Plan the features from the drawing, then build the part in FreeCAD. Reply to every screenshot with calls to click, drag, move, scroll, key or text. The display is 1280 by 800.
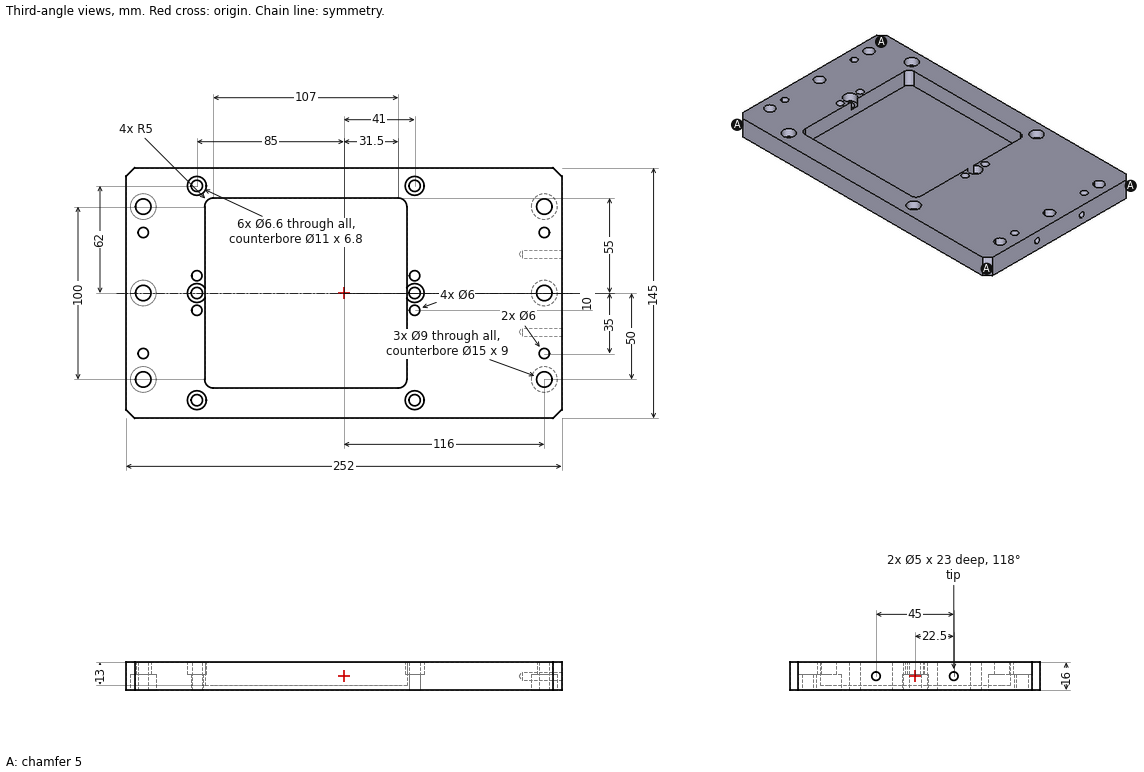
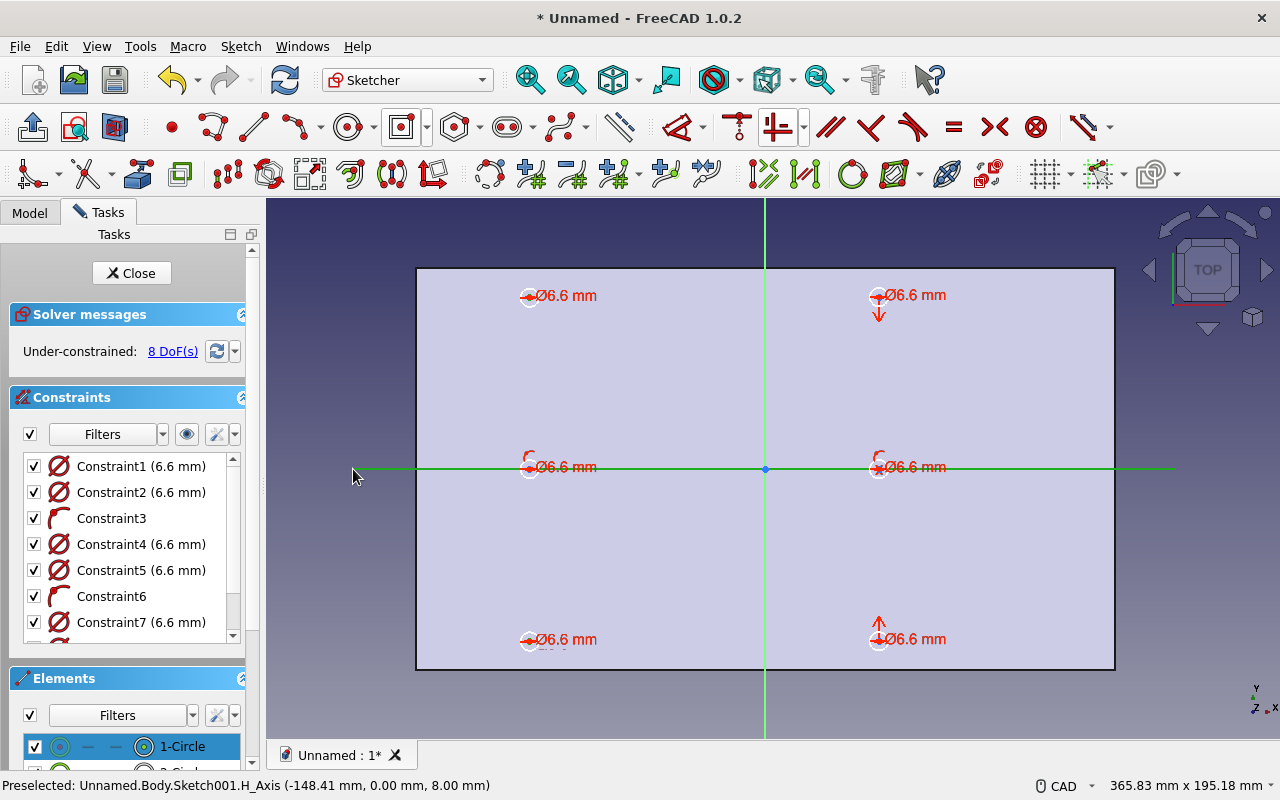
key(s)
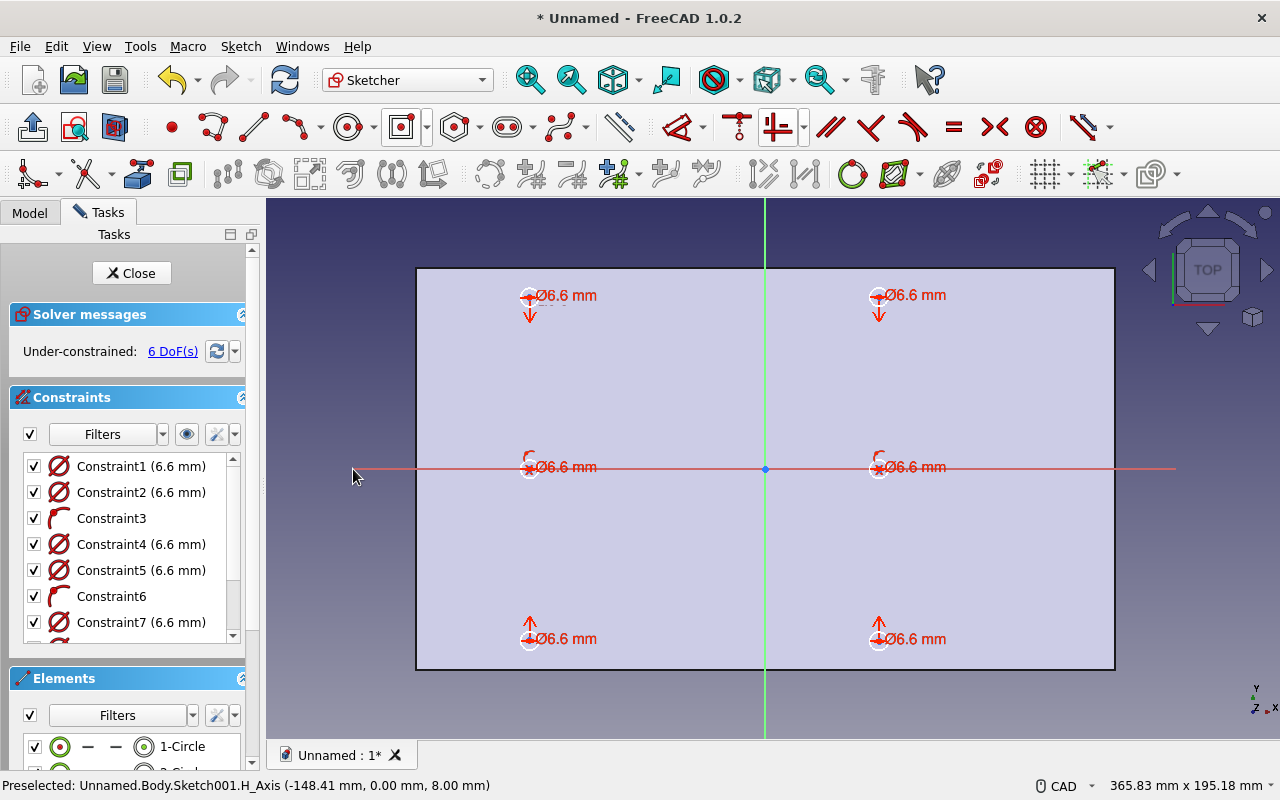
key(d)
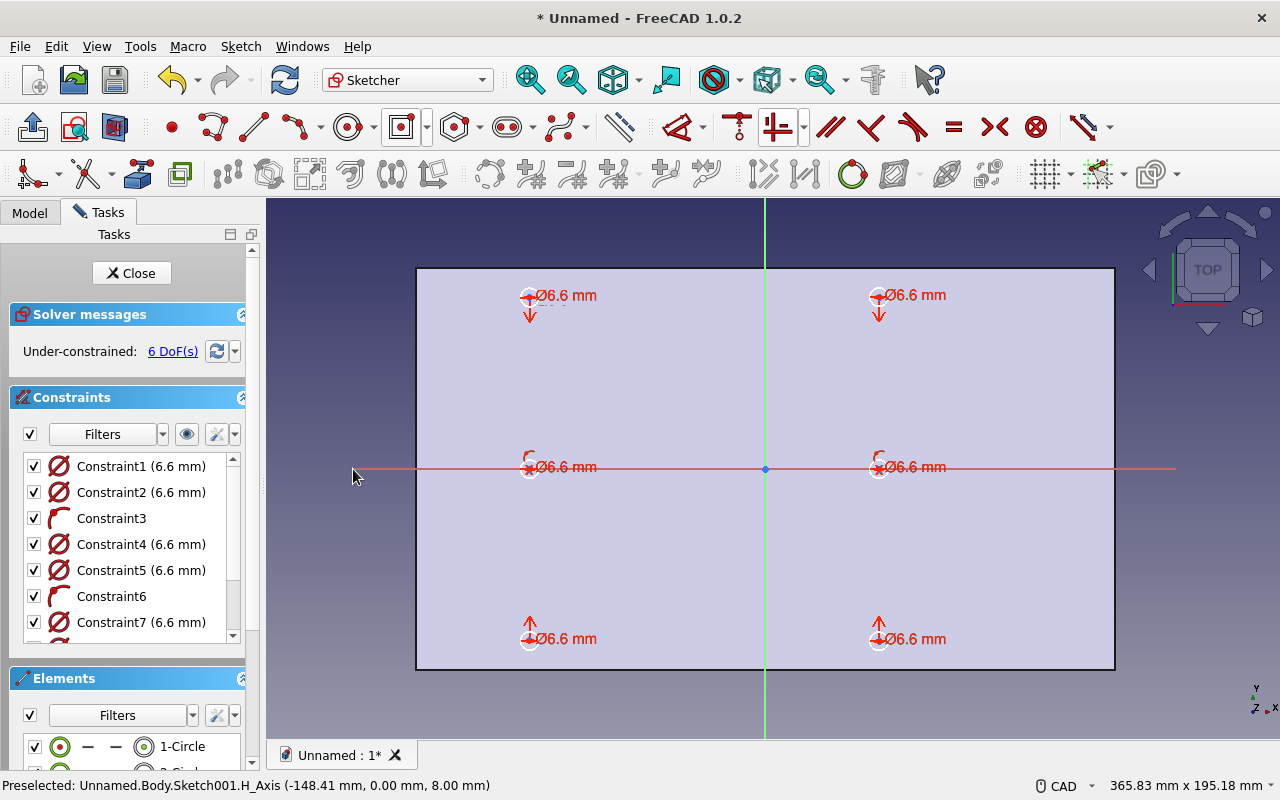
click(530, 298)
click(648, 264)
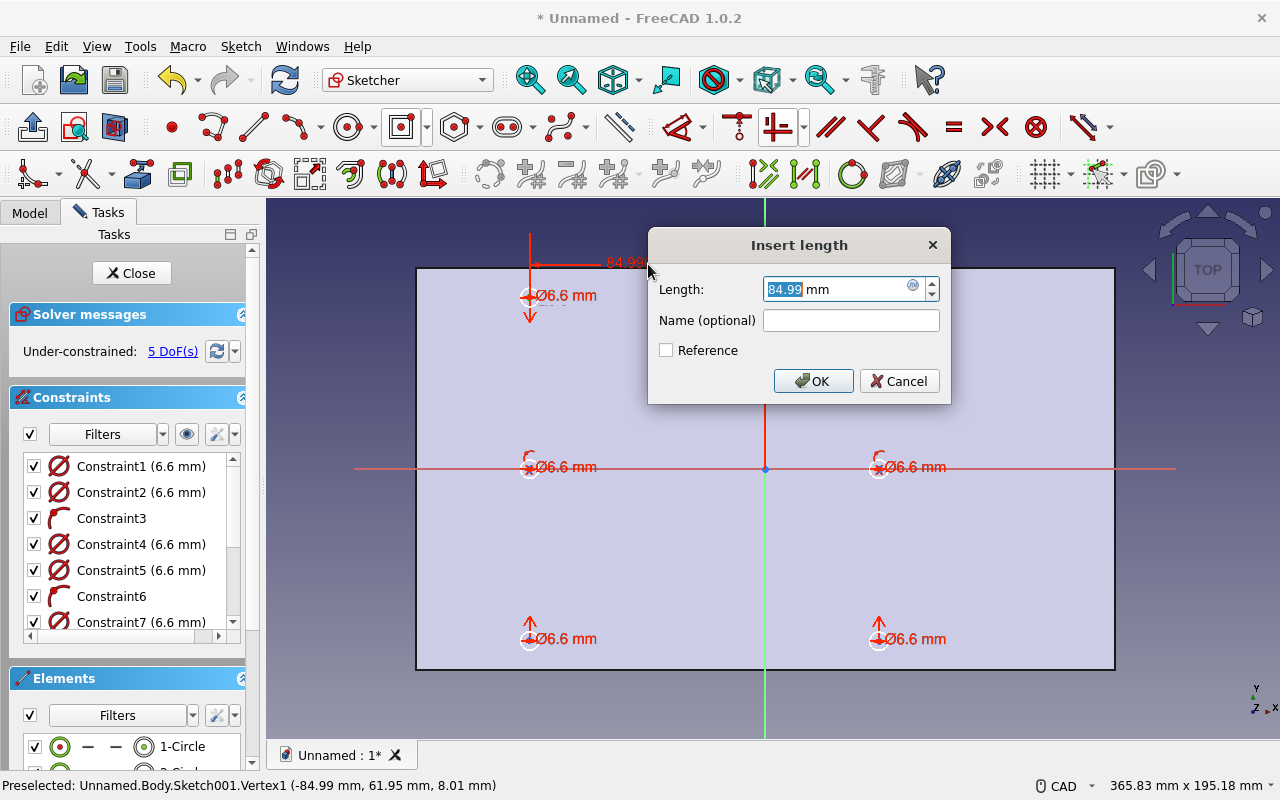
text(85)
key(Return)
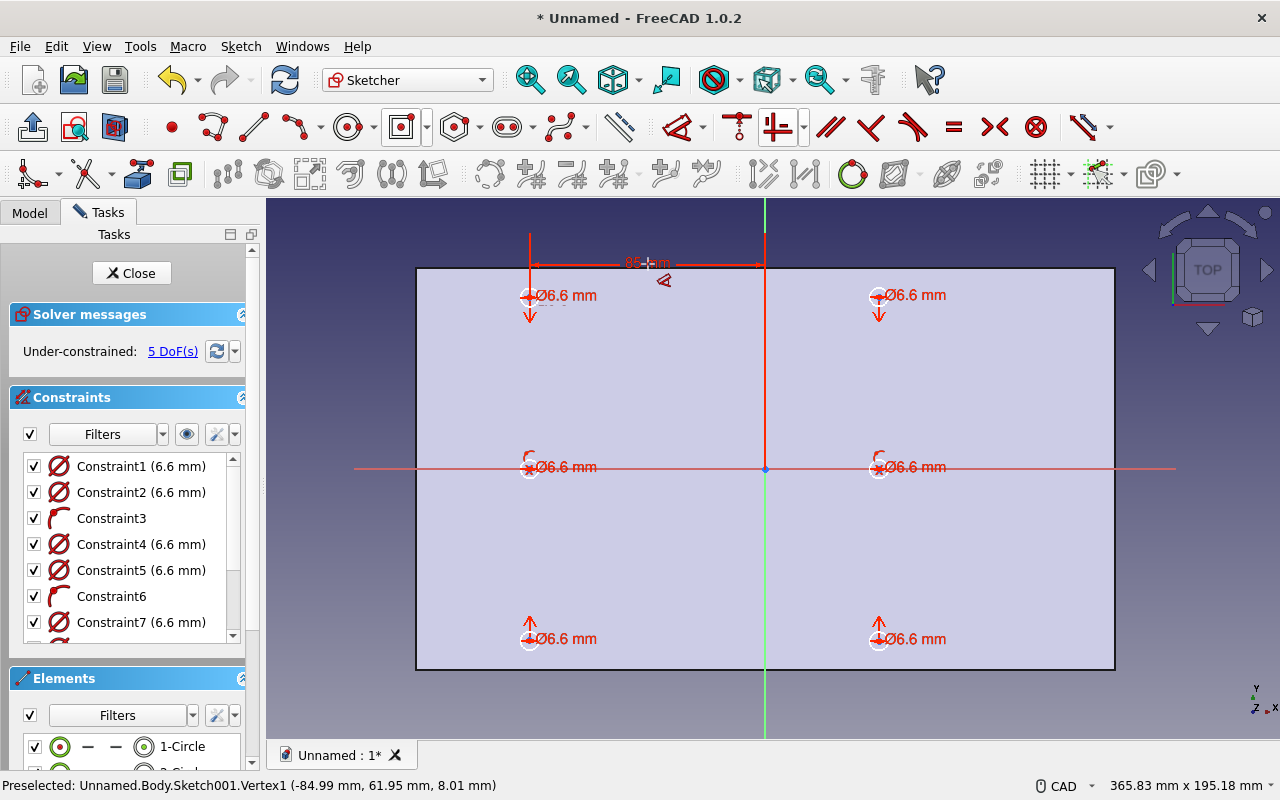
click(530, 298)
click(496, 383)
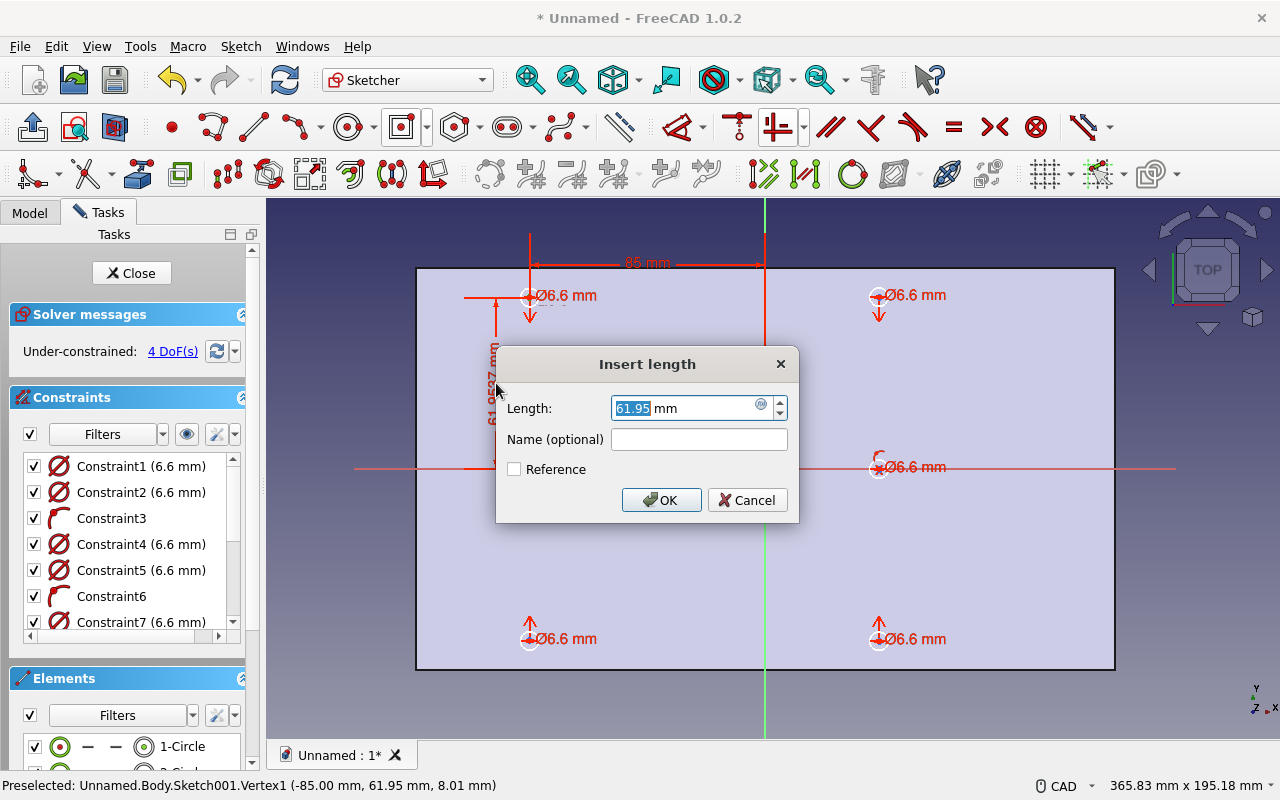
text(62)
key(Return)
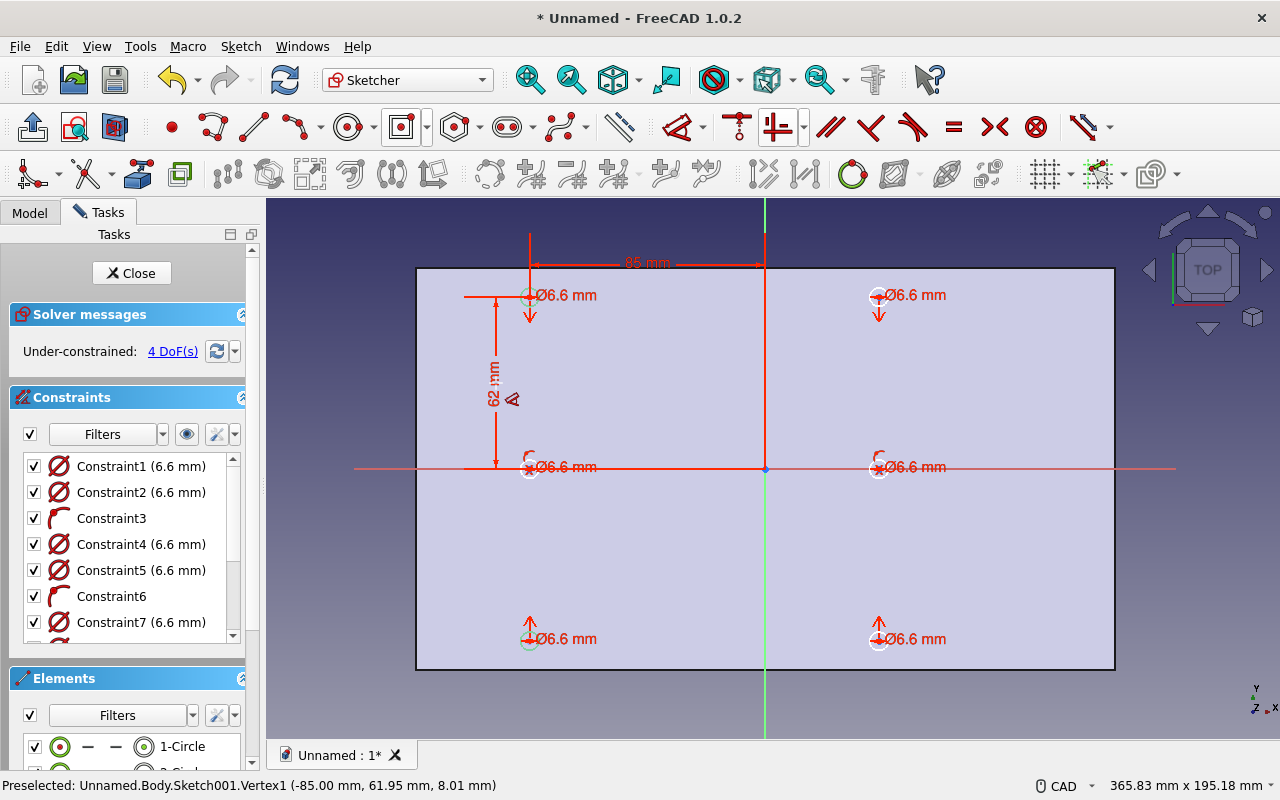
click(530, 469)
click(648, 503)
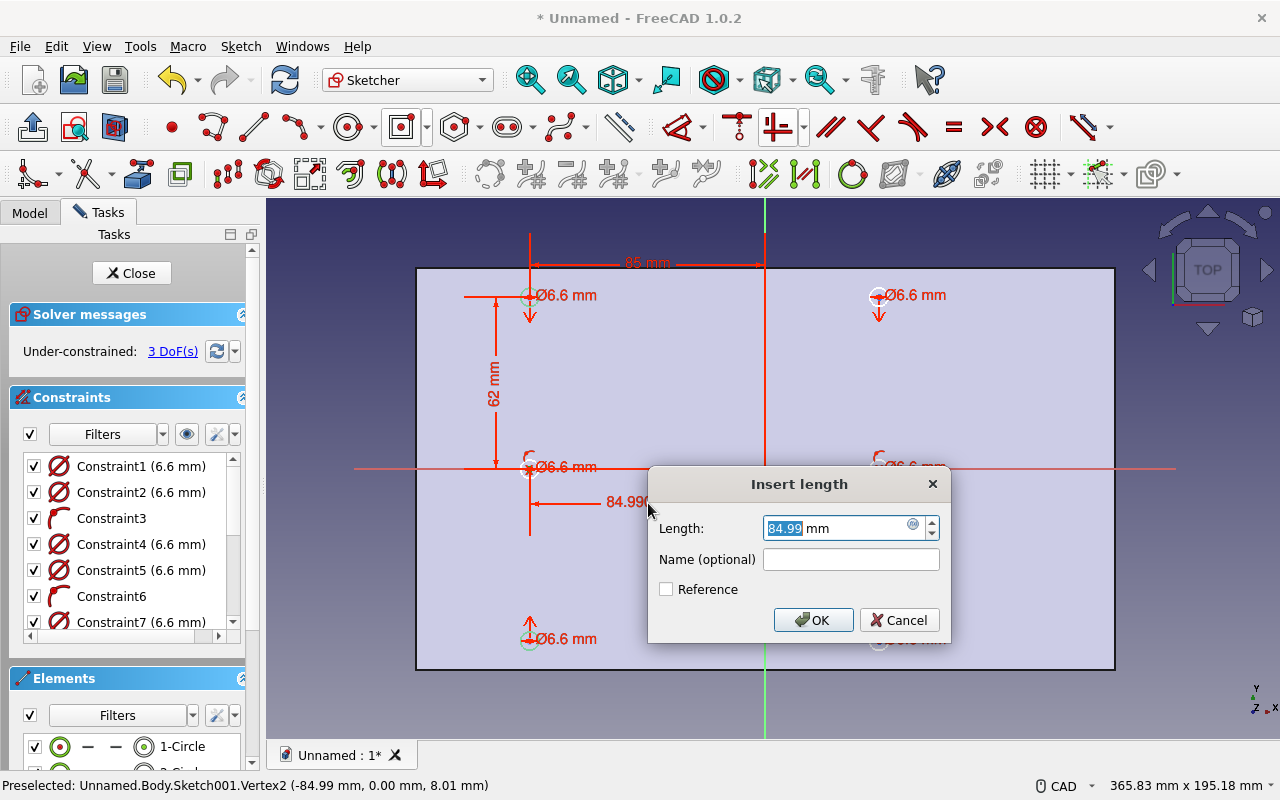
text(85)
key(Return)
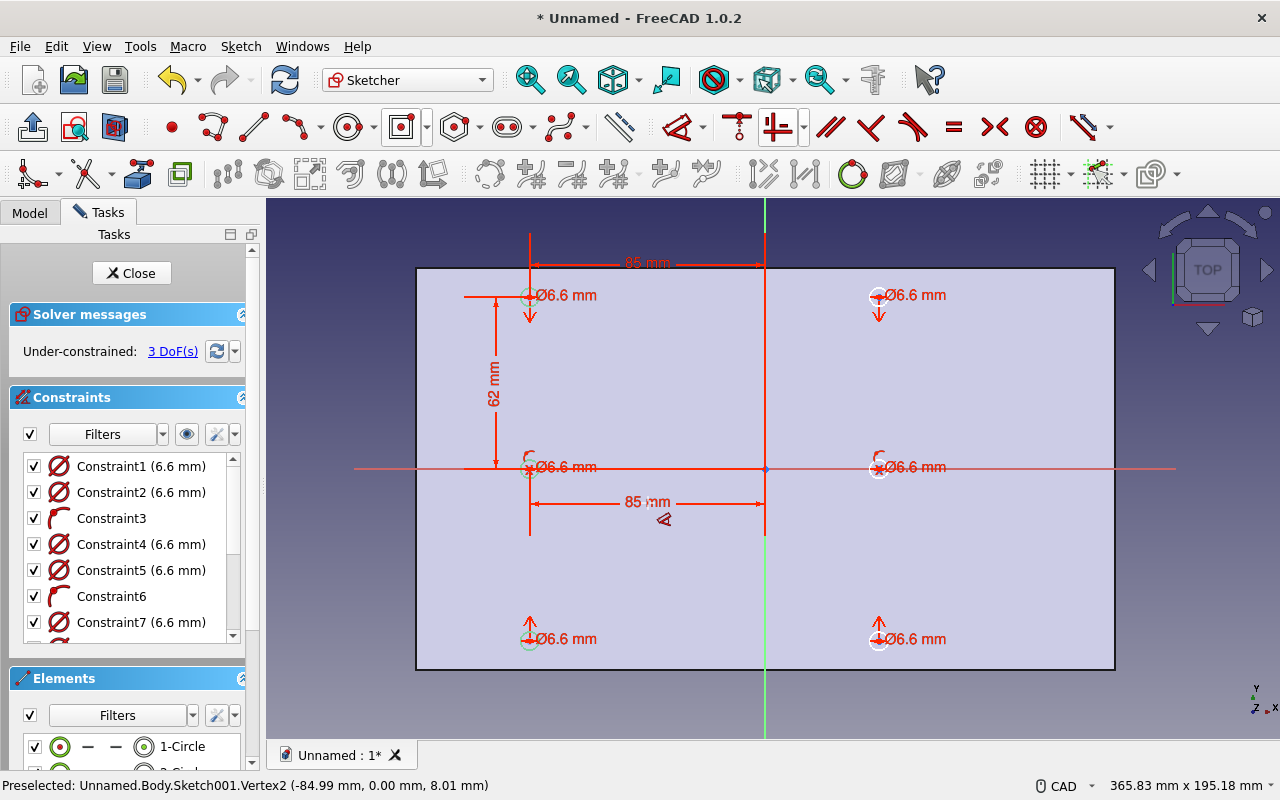
click(879, 297)
click(822, 263)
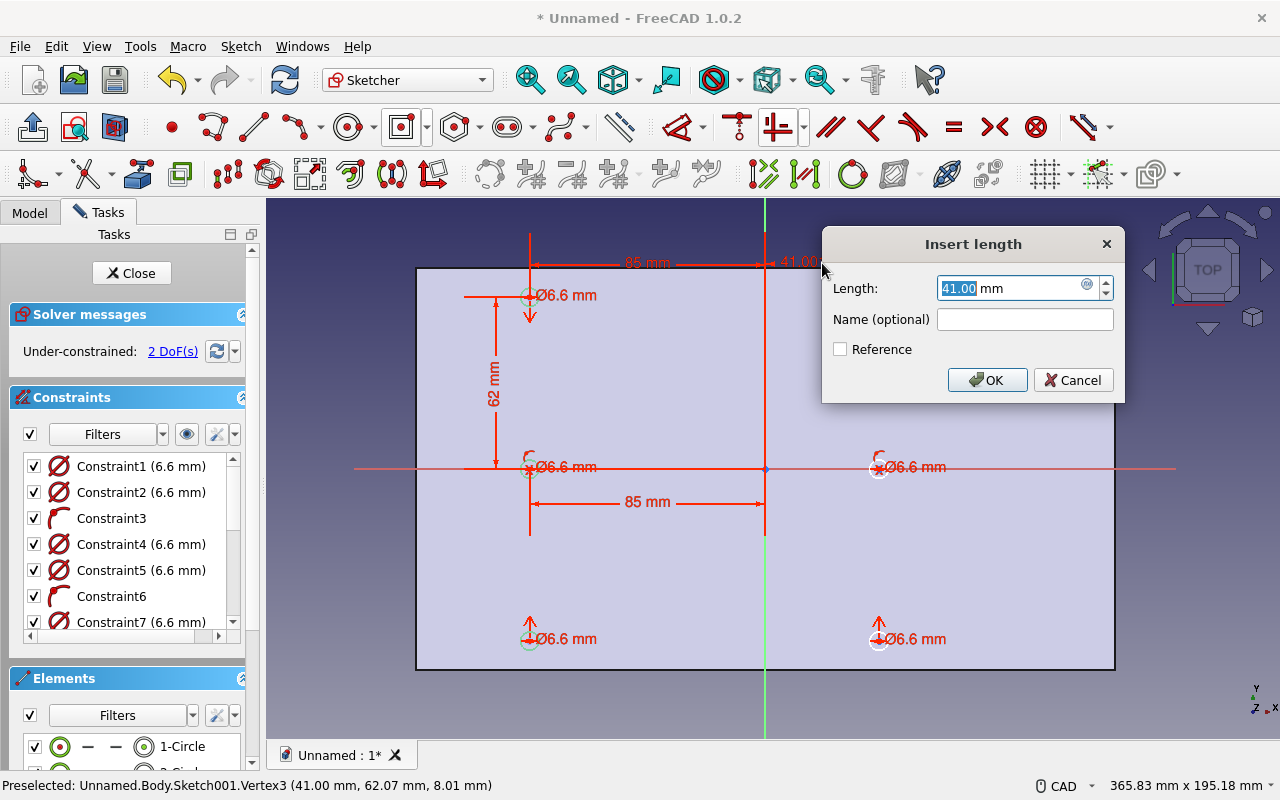
text(41)
key(Return)